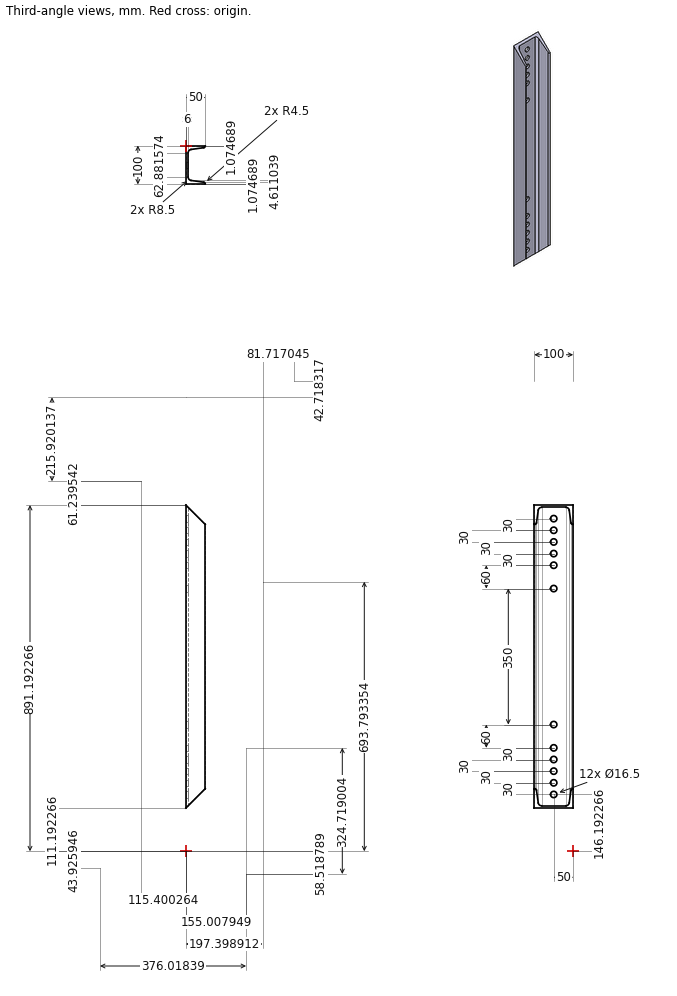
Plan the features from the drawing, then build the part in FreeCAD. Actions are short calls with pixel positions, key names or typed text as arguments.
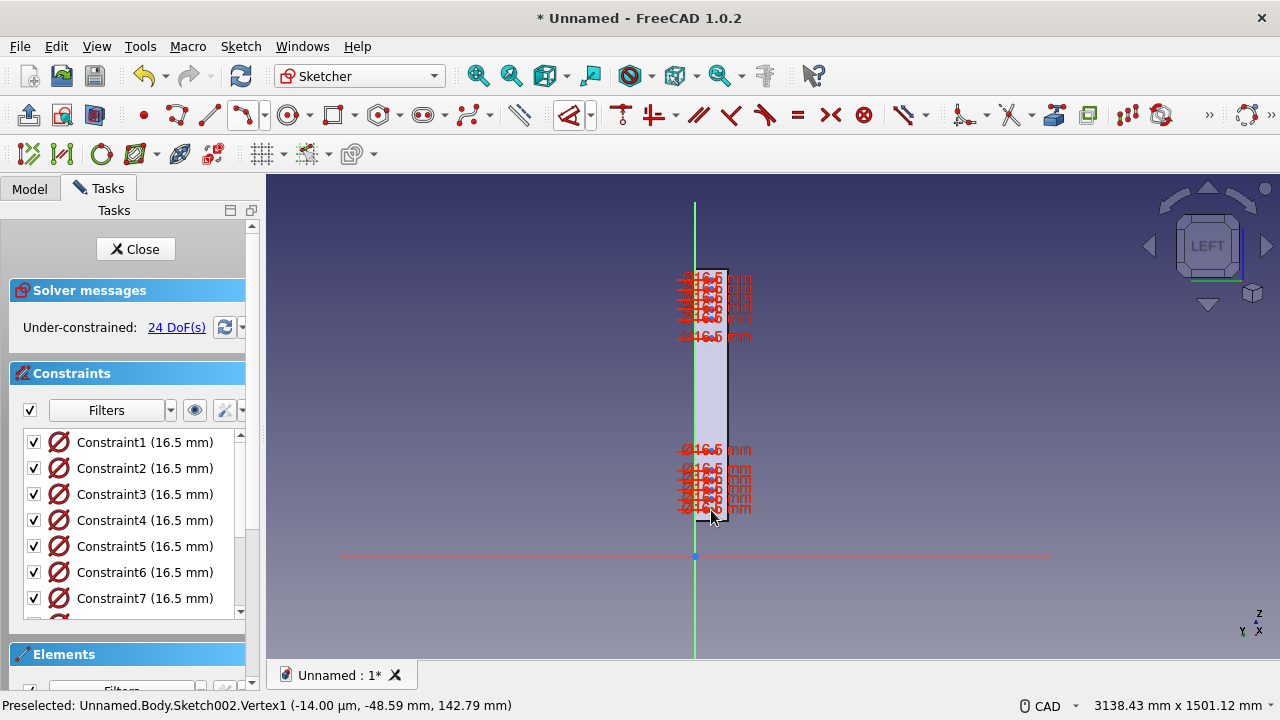
scroll(711, 500, up, 2)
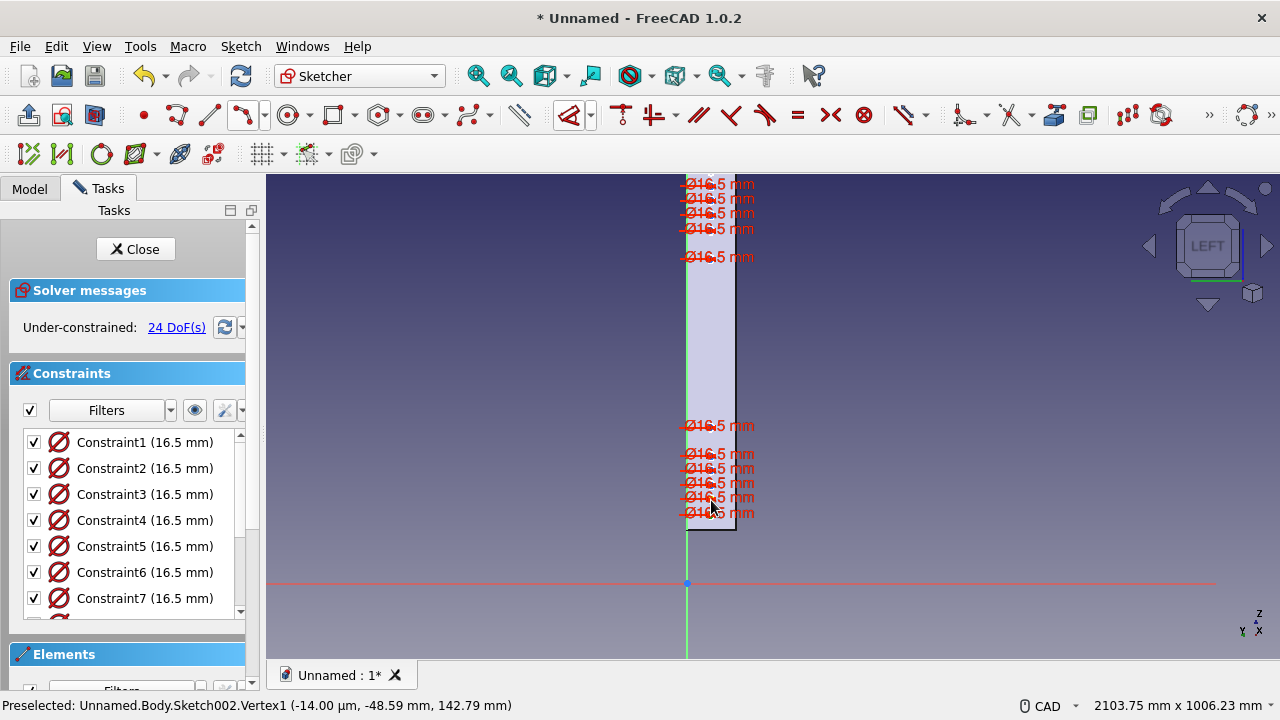
click(711, 499)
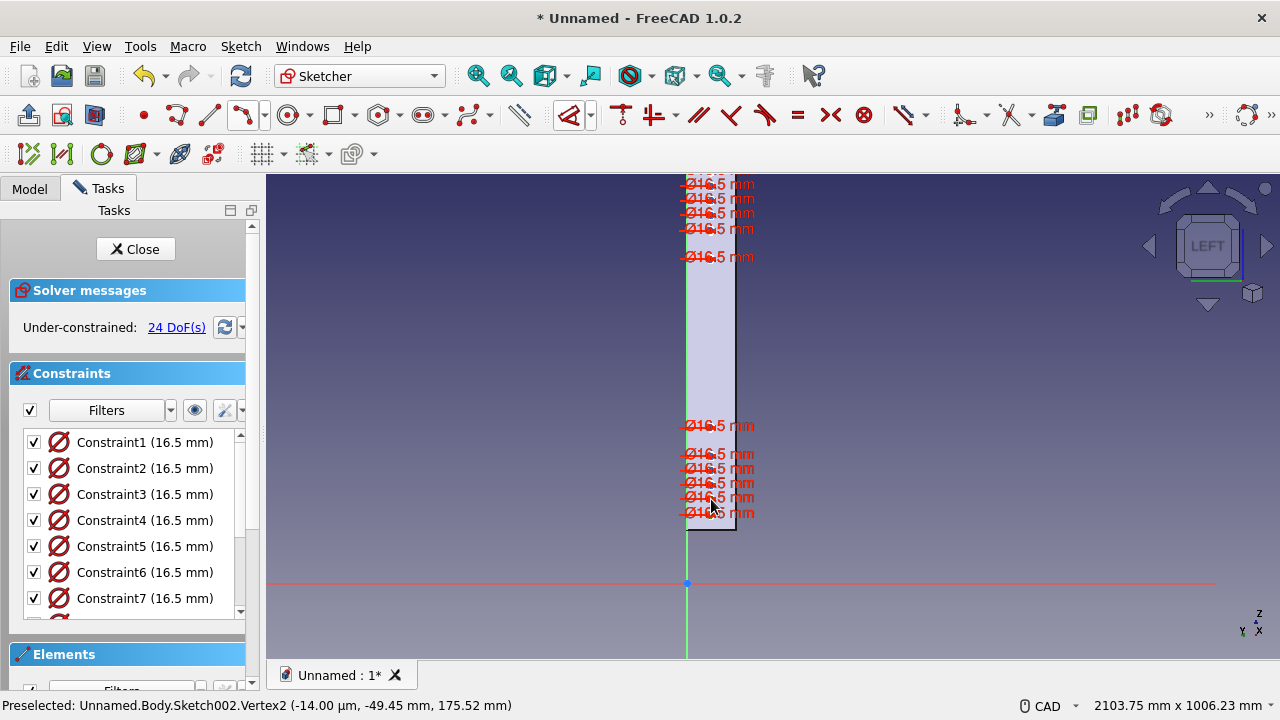
click(676, 116)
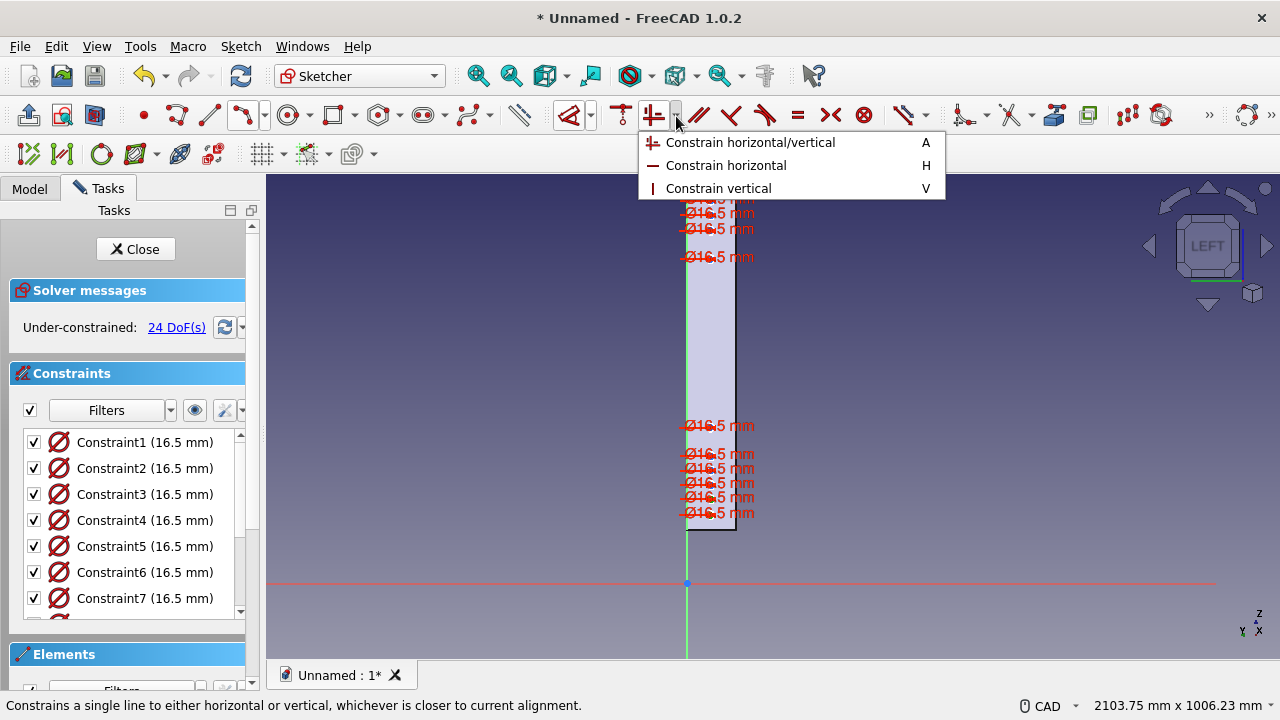
click(792, 188)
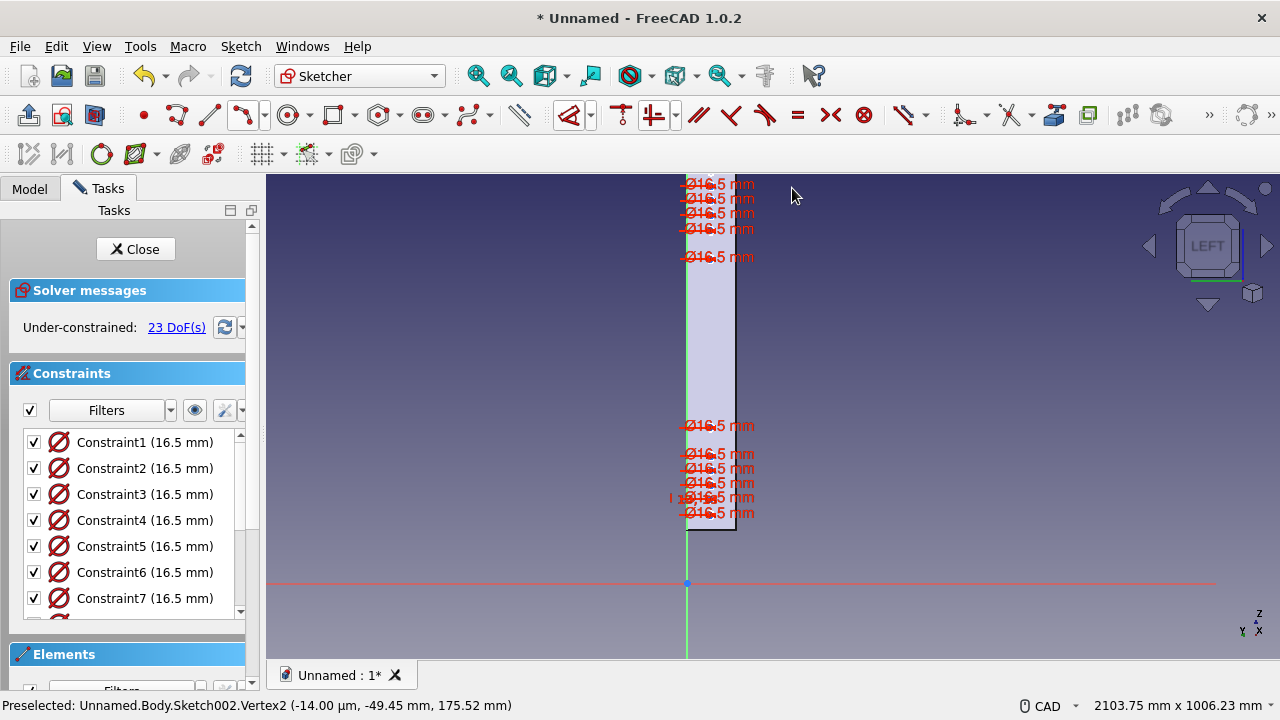
scroll(711, 499, up, 4)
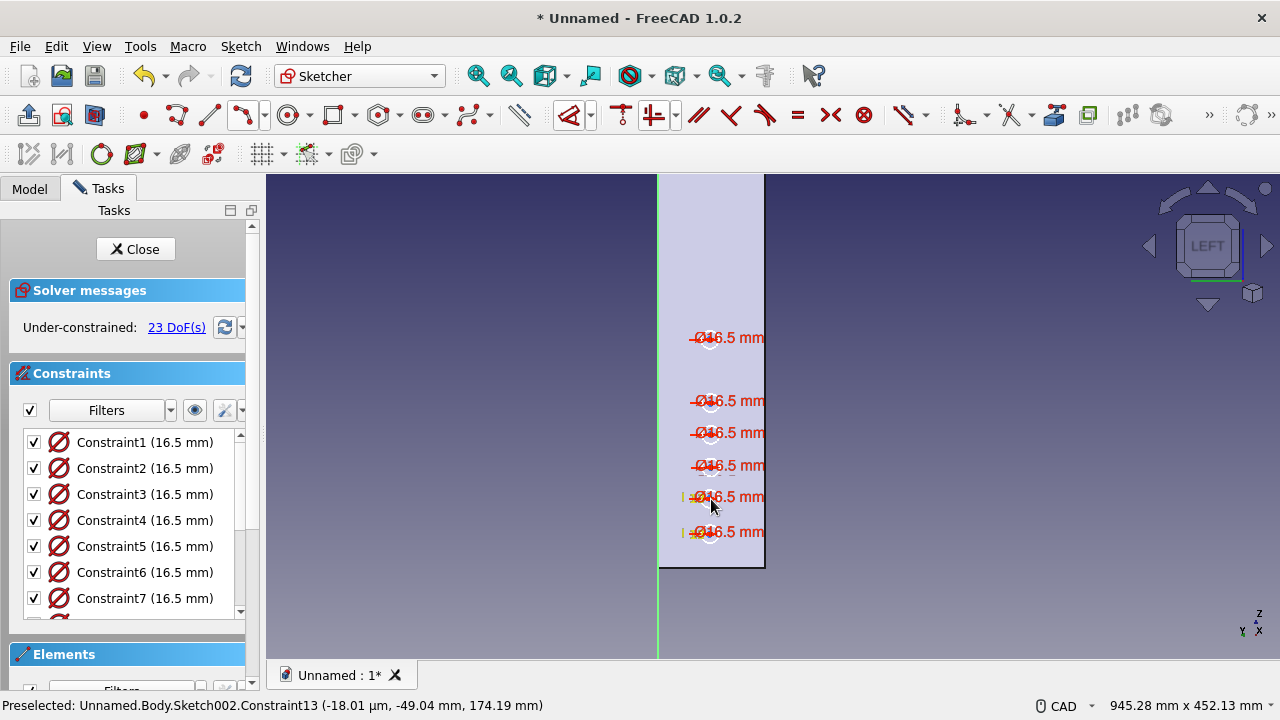
click(710, 499)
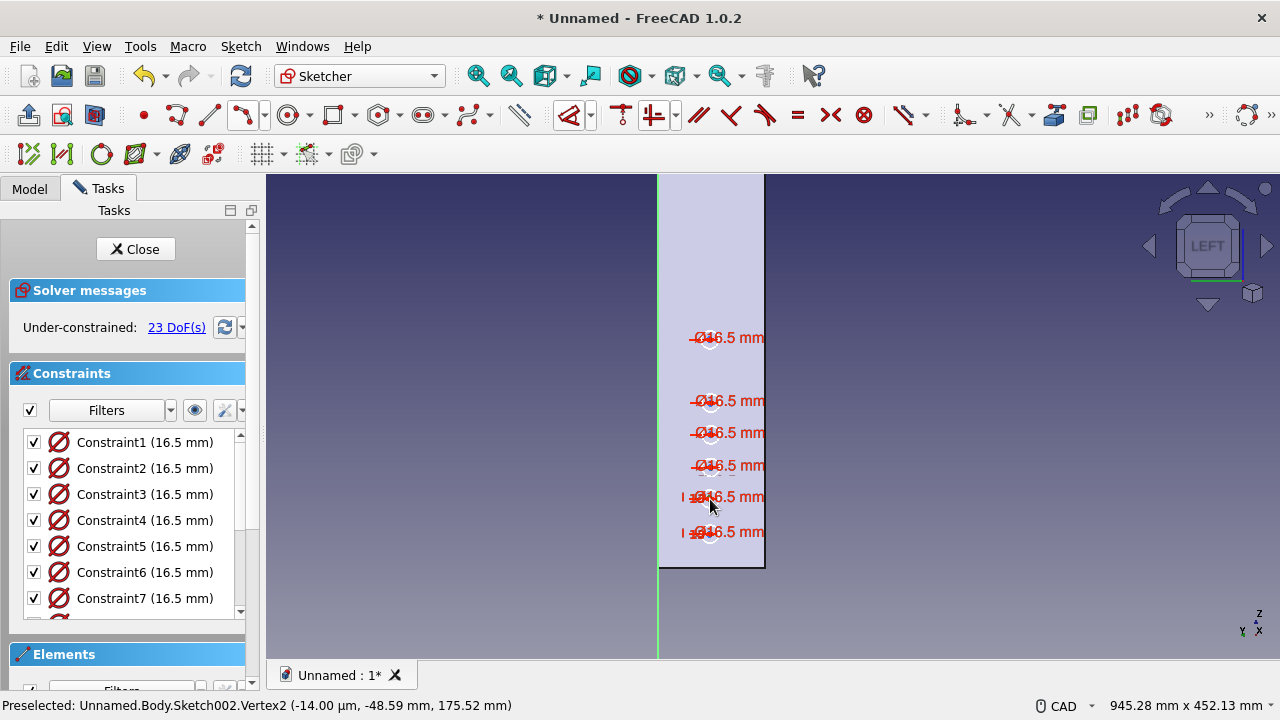
click(711, 468)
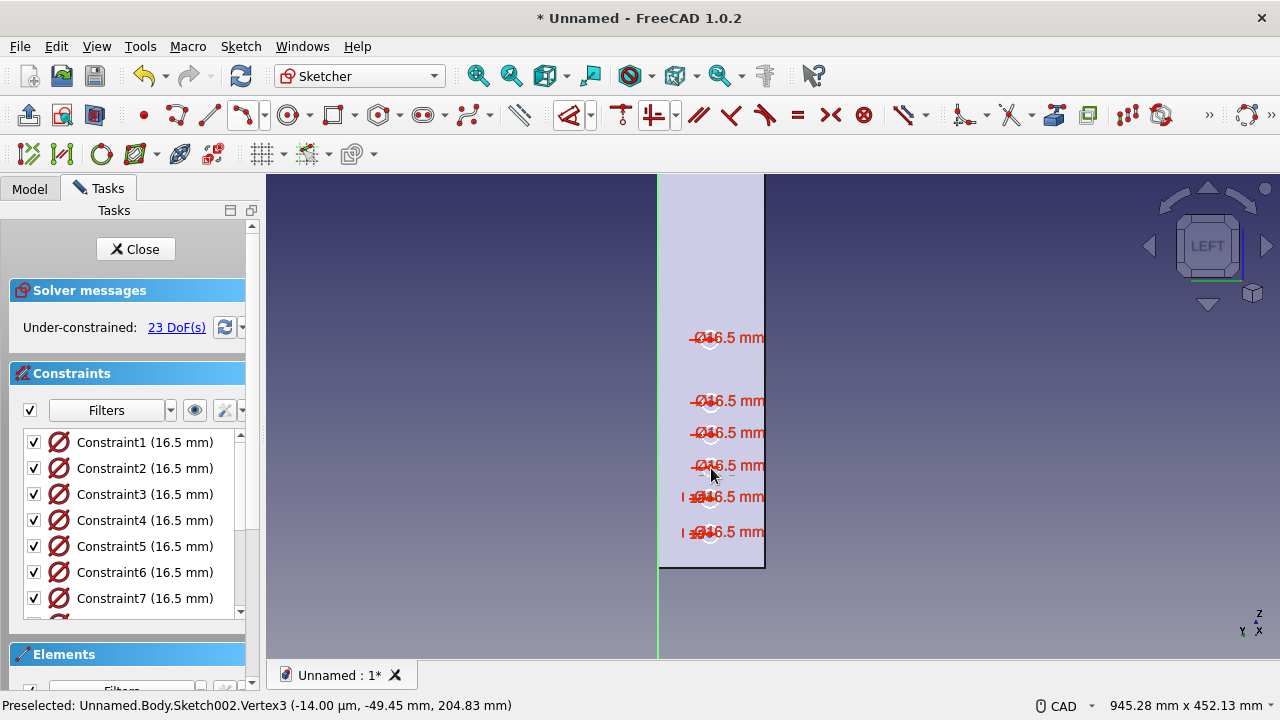
key(v)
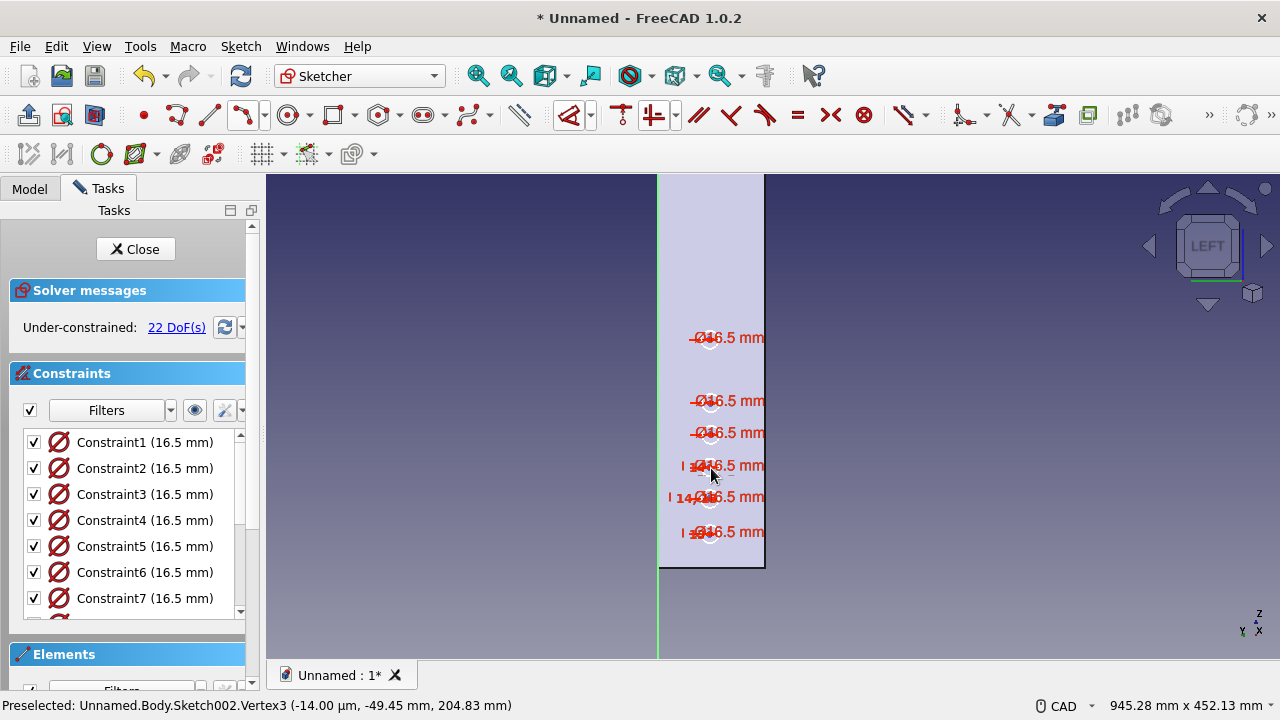
click(710, 468)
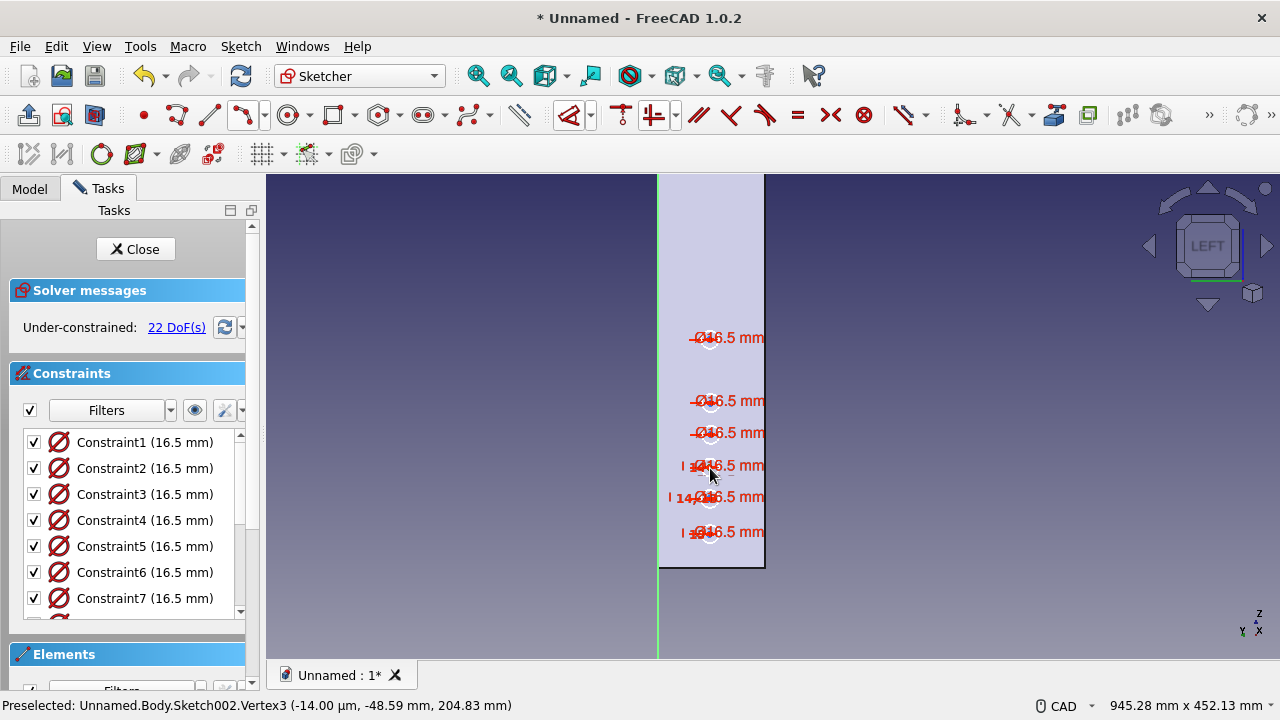
click(711, 435)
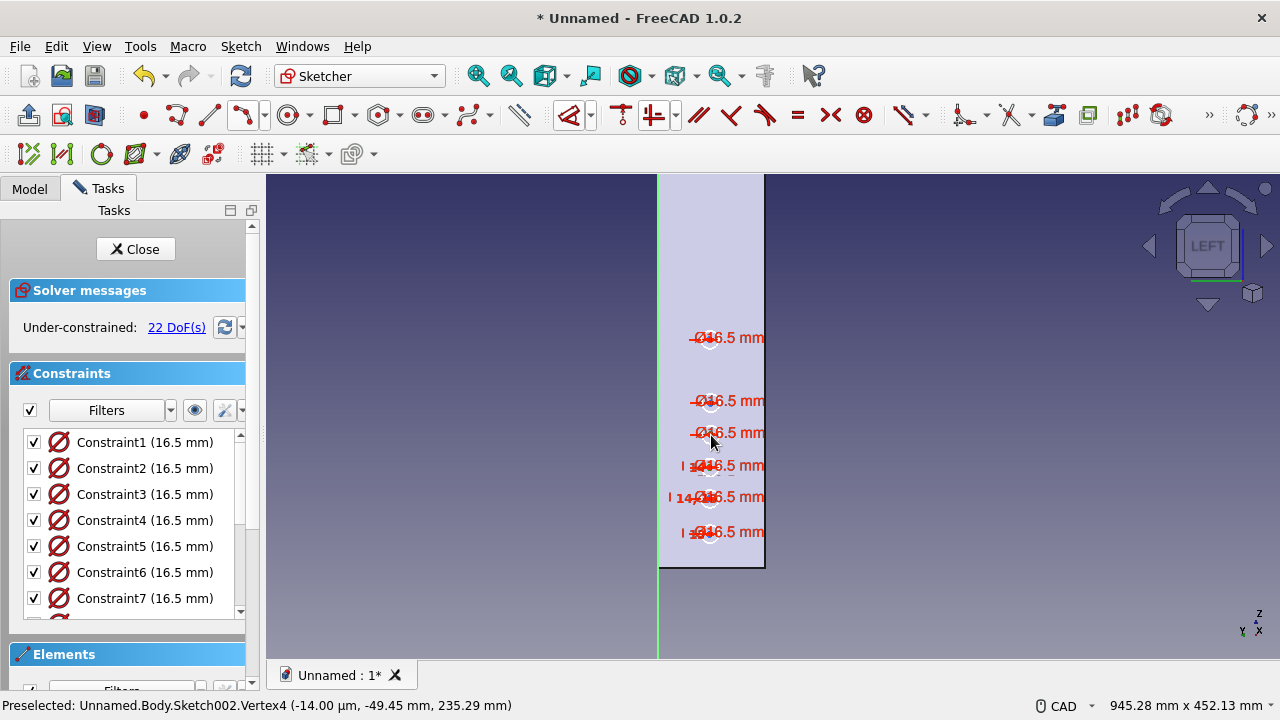
key(v)